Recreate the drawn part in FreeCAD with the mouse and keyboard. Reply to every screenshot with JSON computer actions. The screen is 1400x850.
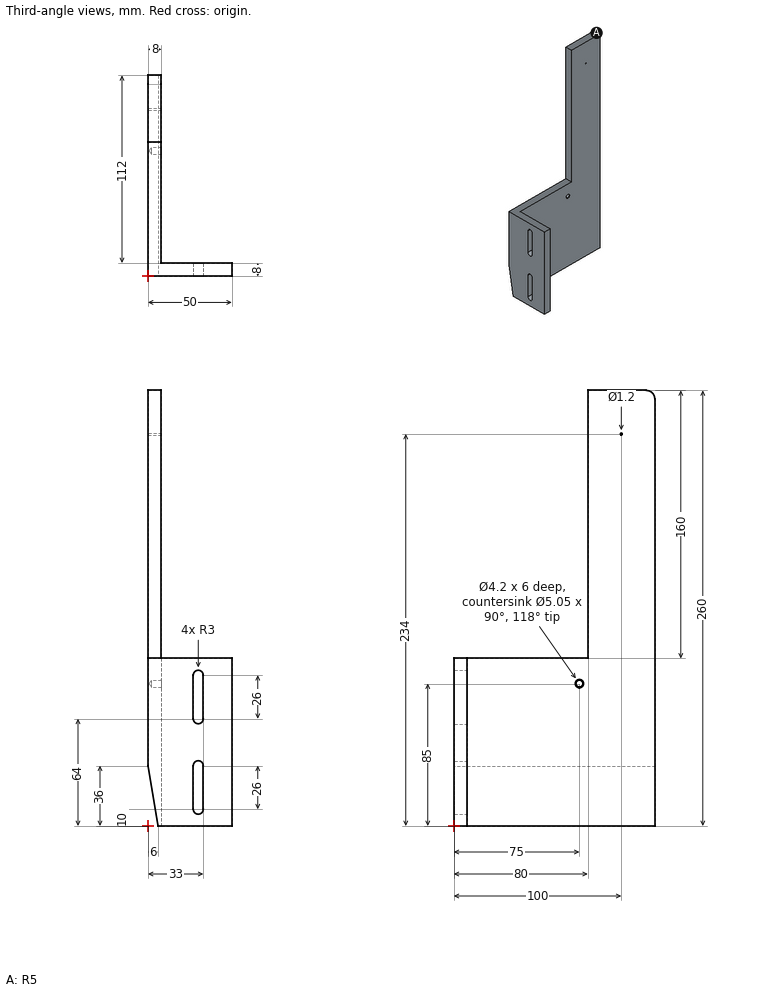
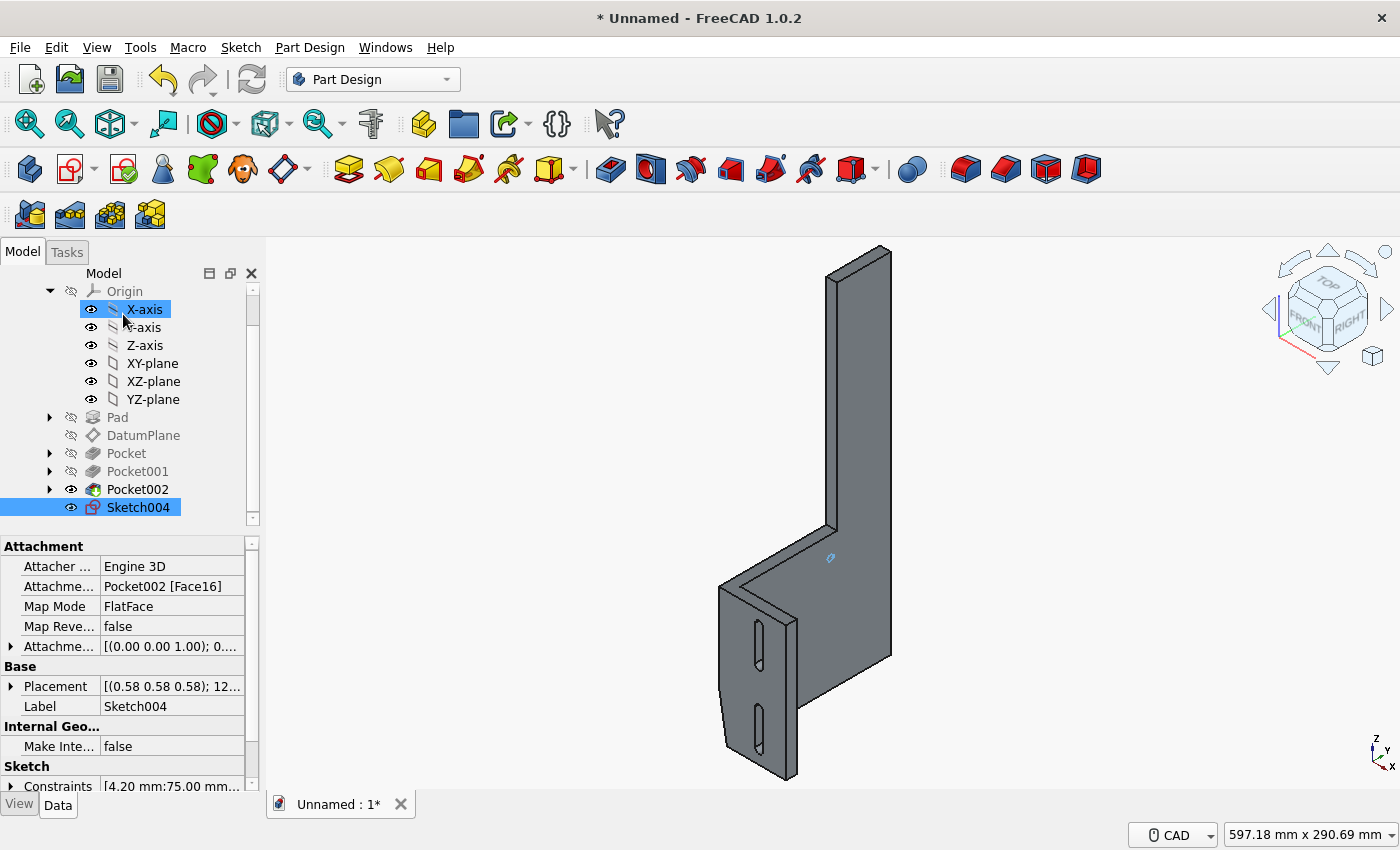
{"action": "left_click", "coordinate": [652, 170]}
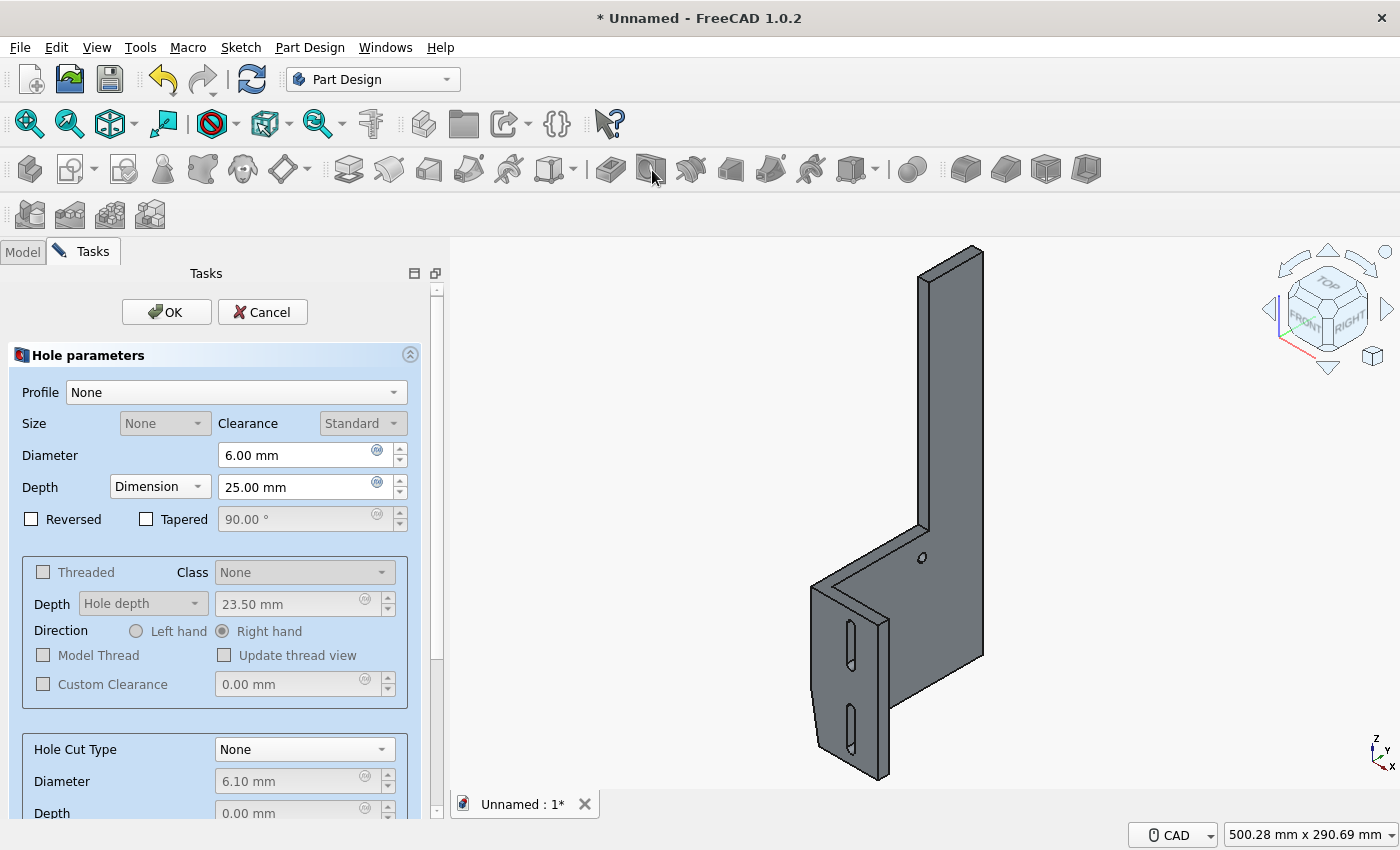
{"action": "triple_click", "coordinate": [305, 455]}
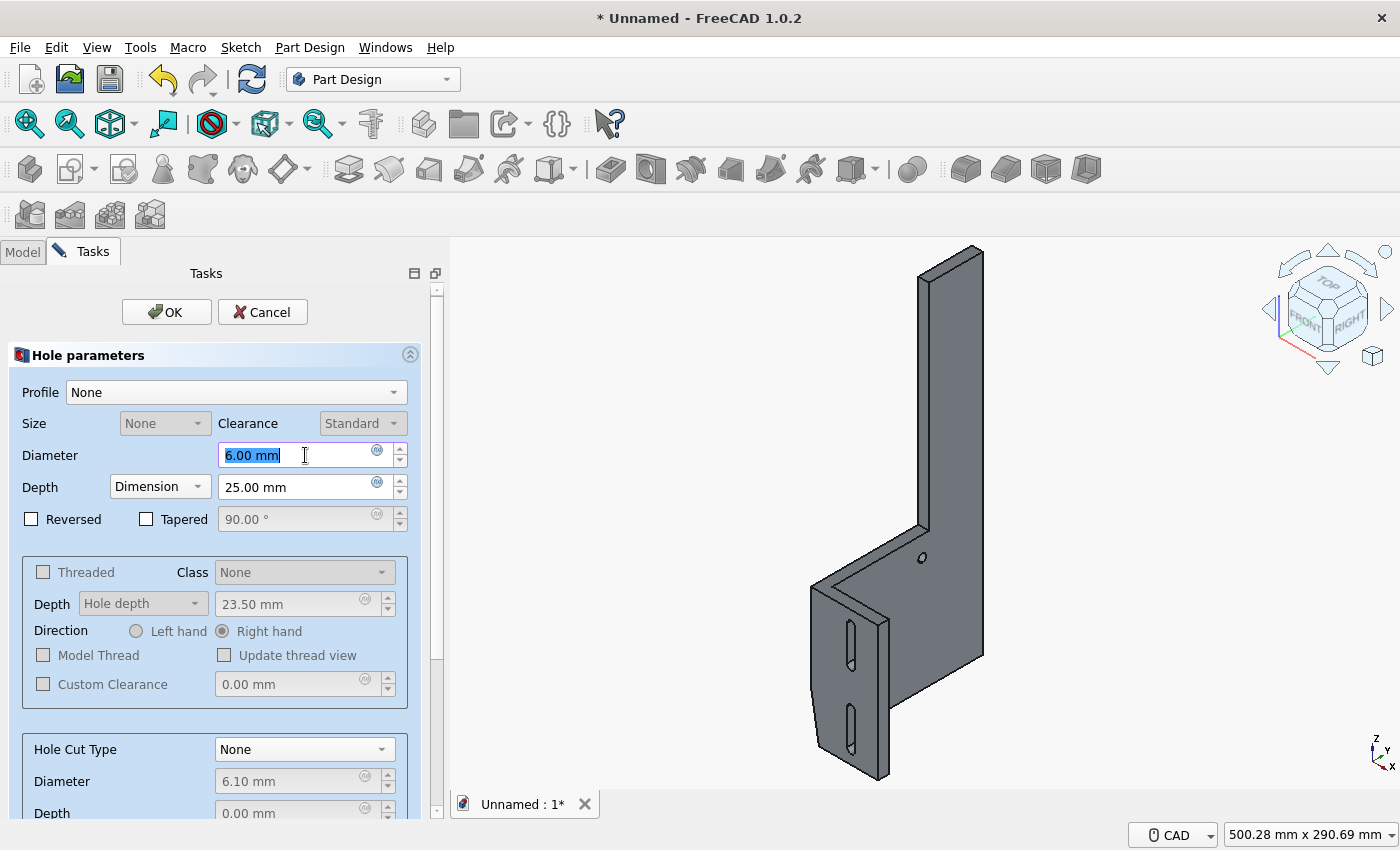
{"action": "type", "text": "4.2"}
{"action": "key", "text": "Tab"}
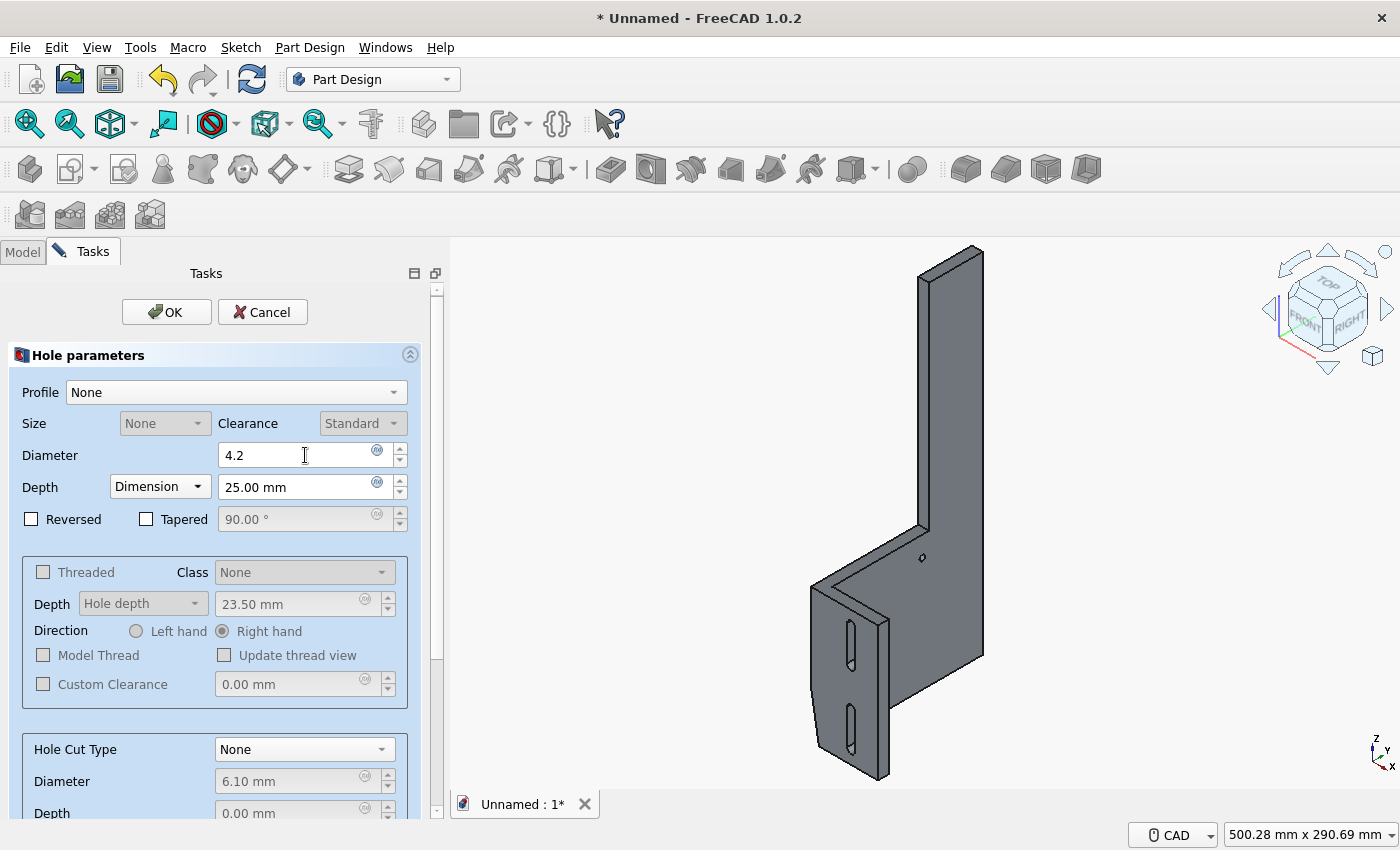
{"action": "triple_click", "coordinate": [305, 487]}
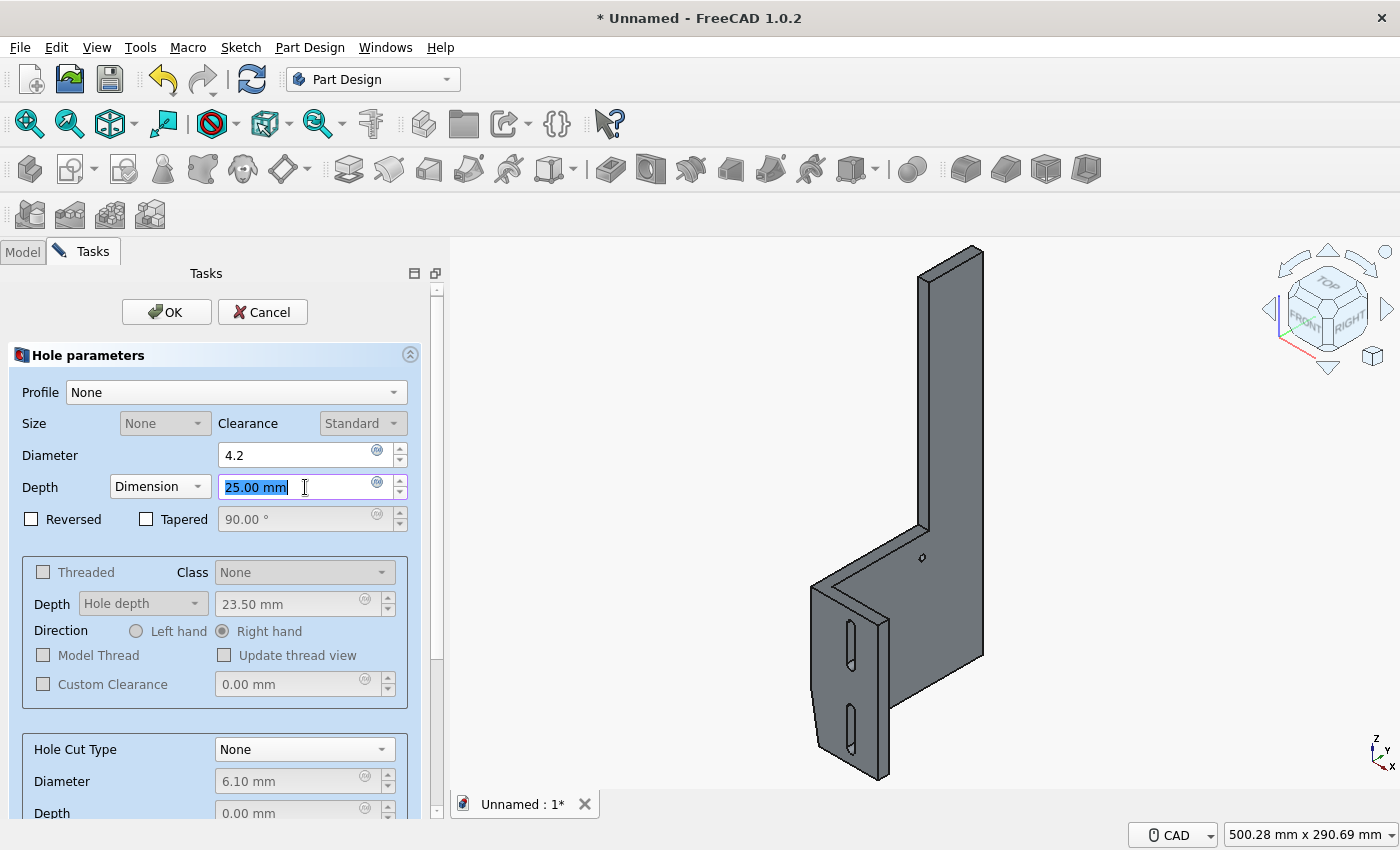
{"action": "type", "text": "6"}
{"action": "key", "text": "Tab"}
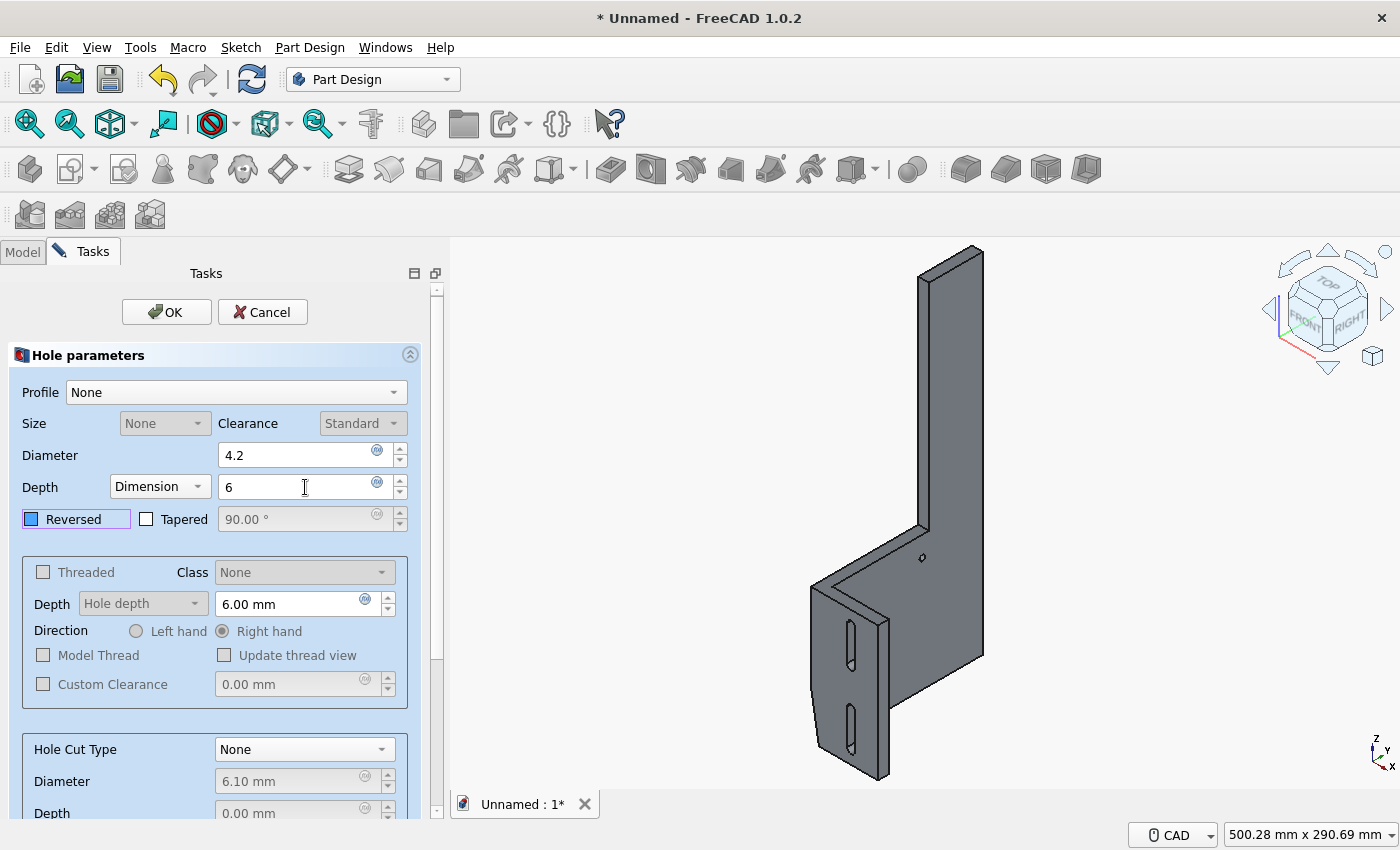
{"action": "left_click", "coordinate": [306, 750]}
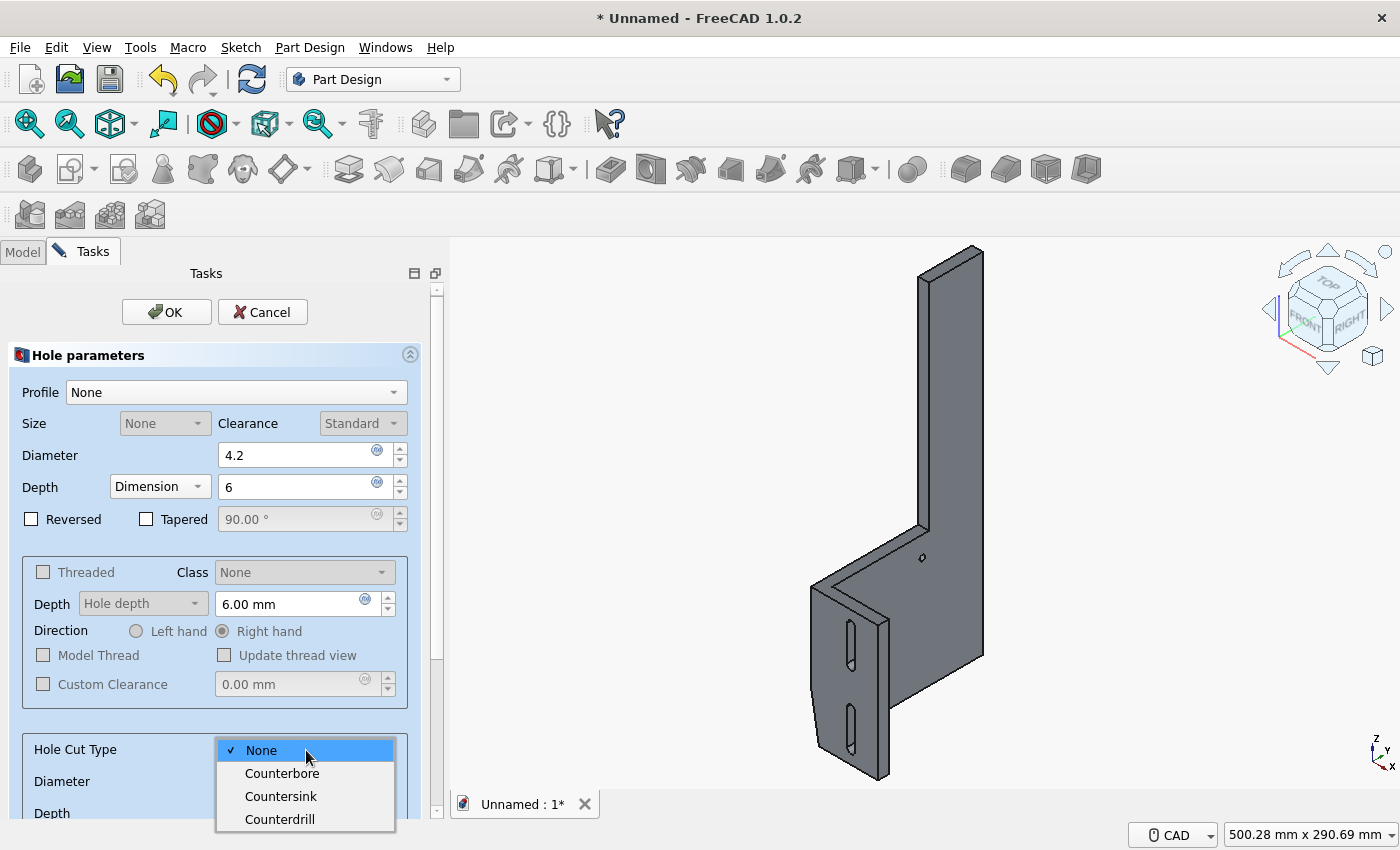
{"action": "left_click", "coordinate": [304, 796]}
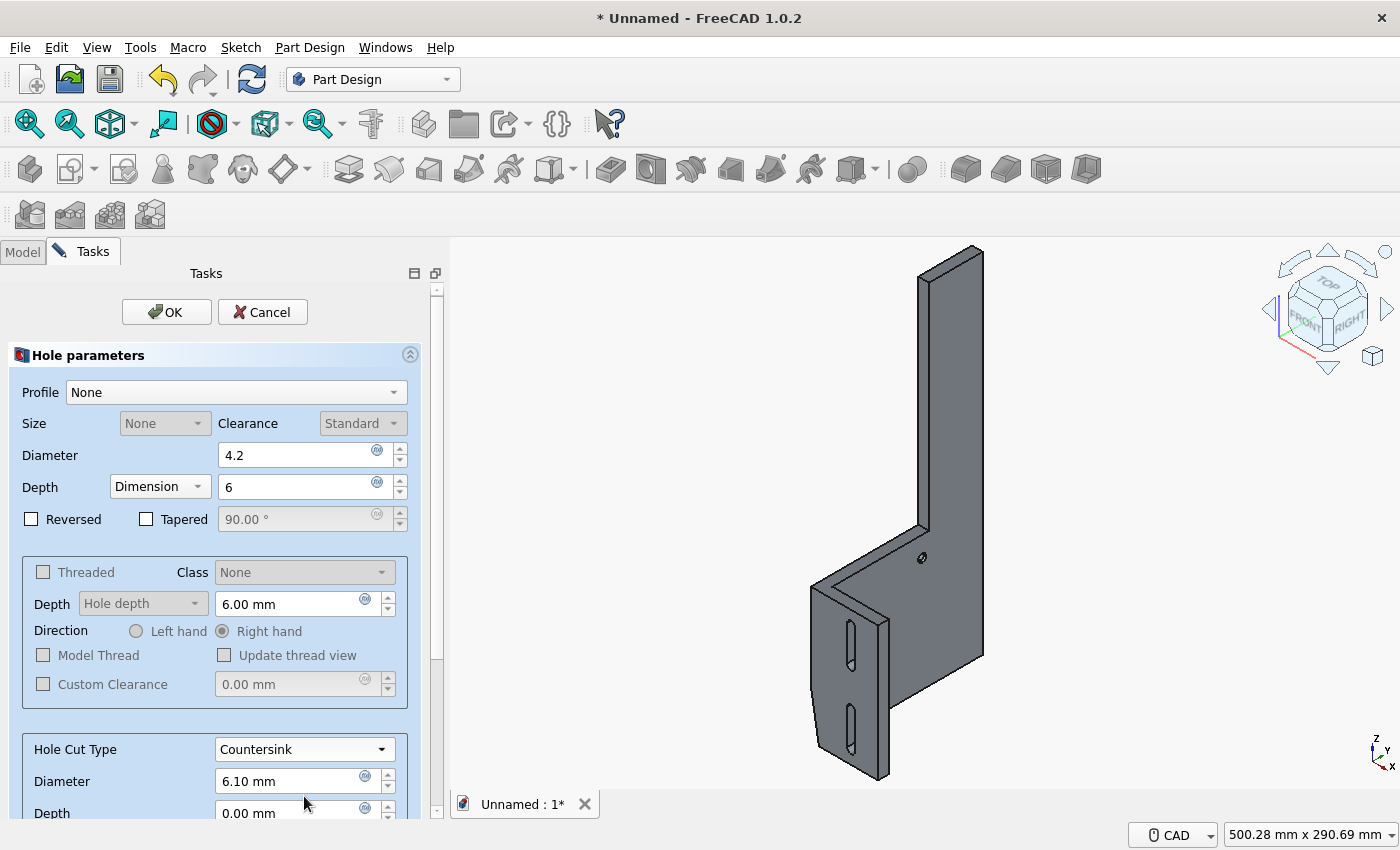
{"action": "triple_click", "coordinate": [298, 781]}